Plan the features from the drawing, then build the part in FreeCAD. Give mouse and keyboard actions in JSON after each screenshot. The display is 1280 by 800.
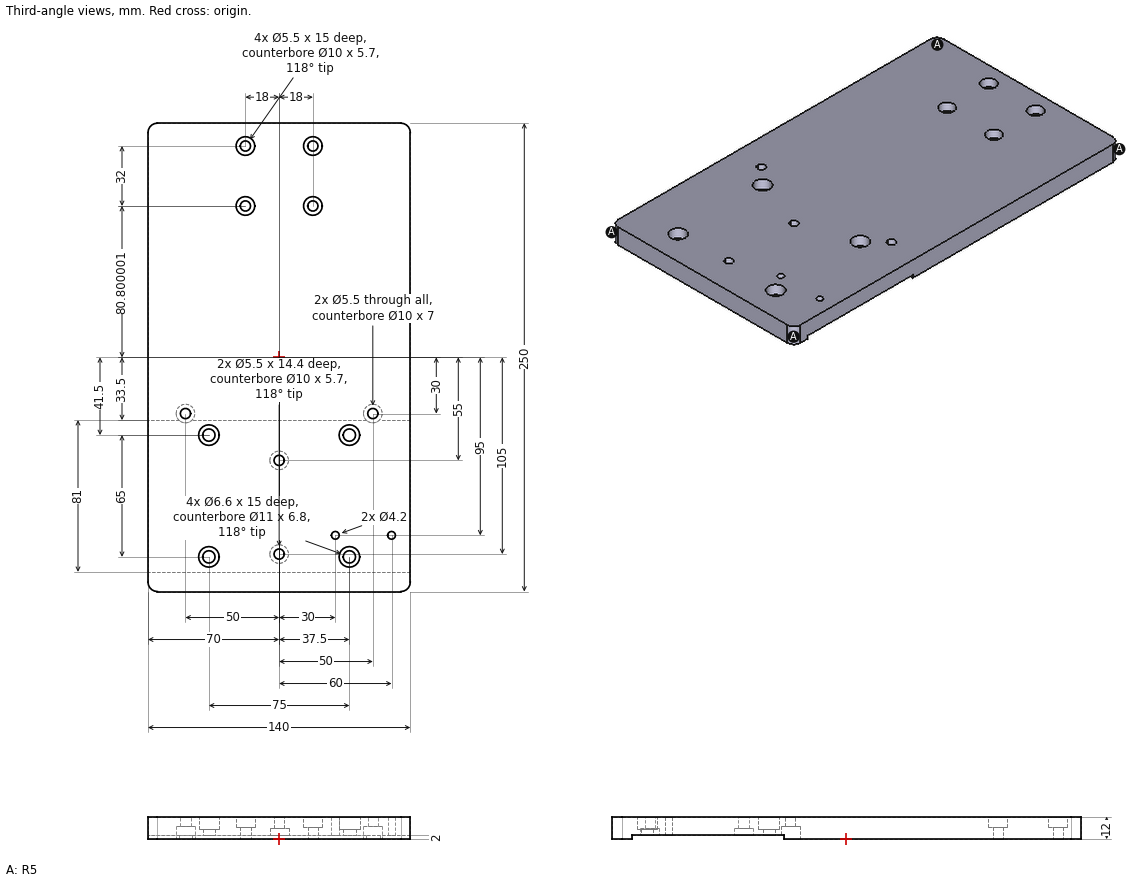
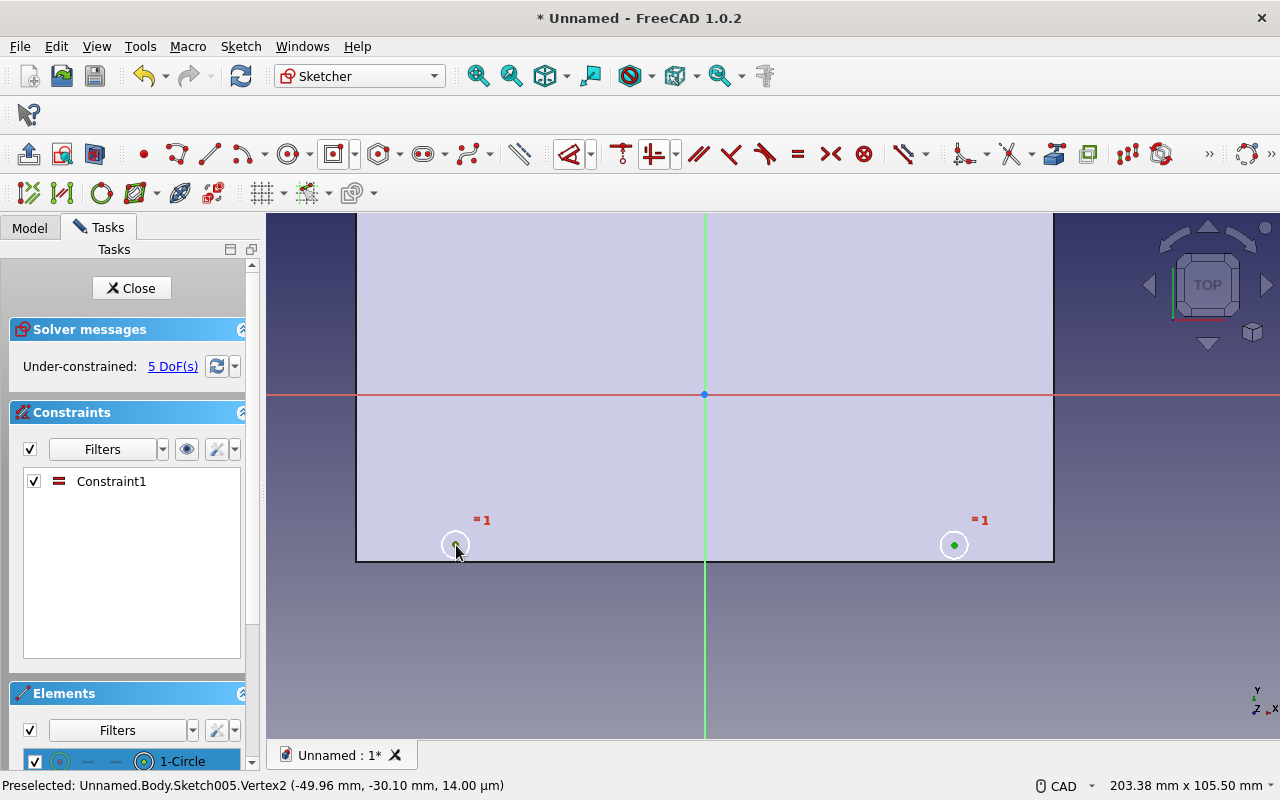
{"action": "key", "text": "h"}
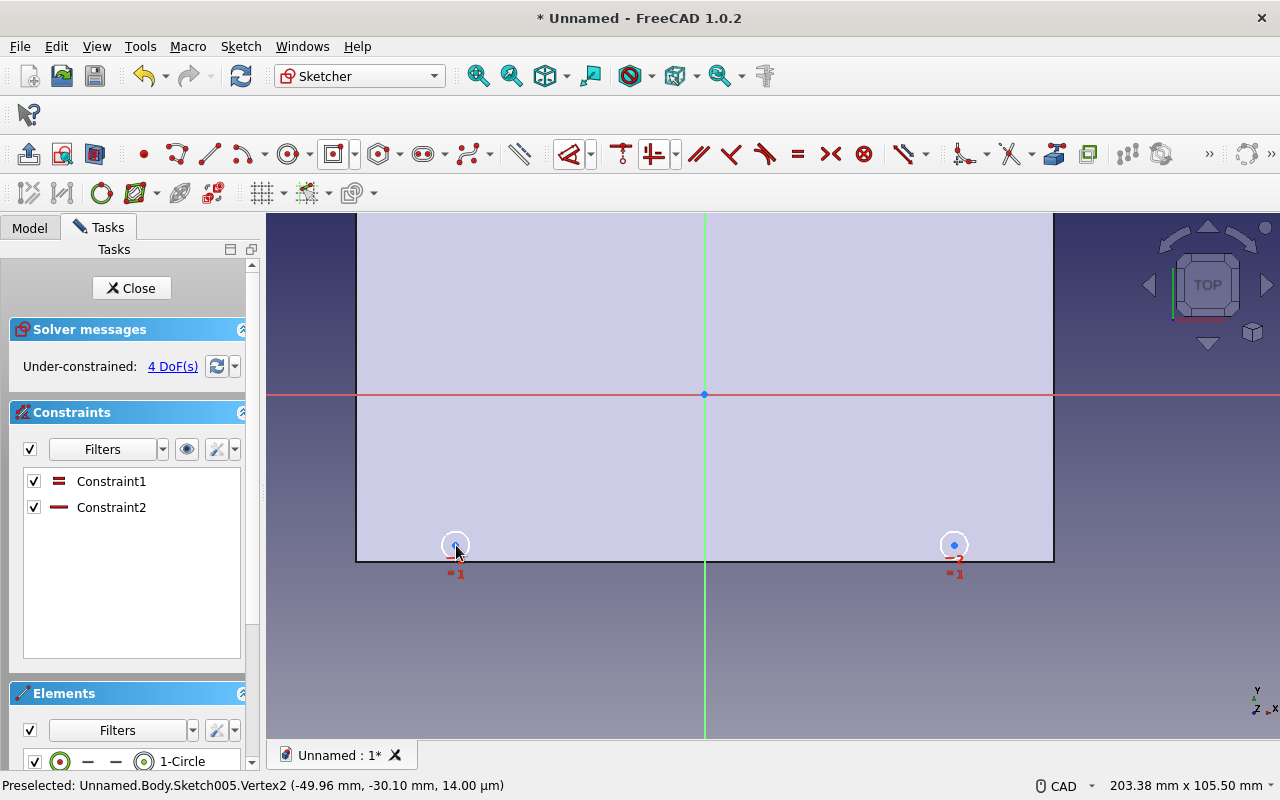
{"action": "scroll", "coordinate": [964, 535], "scroll_direction": "up", "scroll_amount": 2}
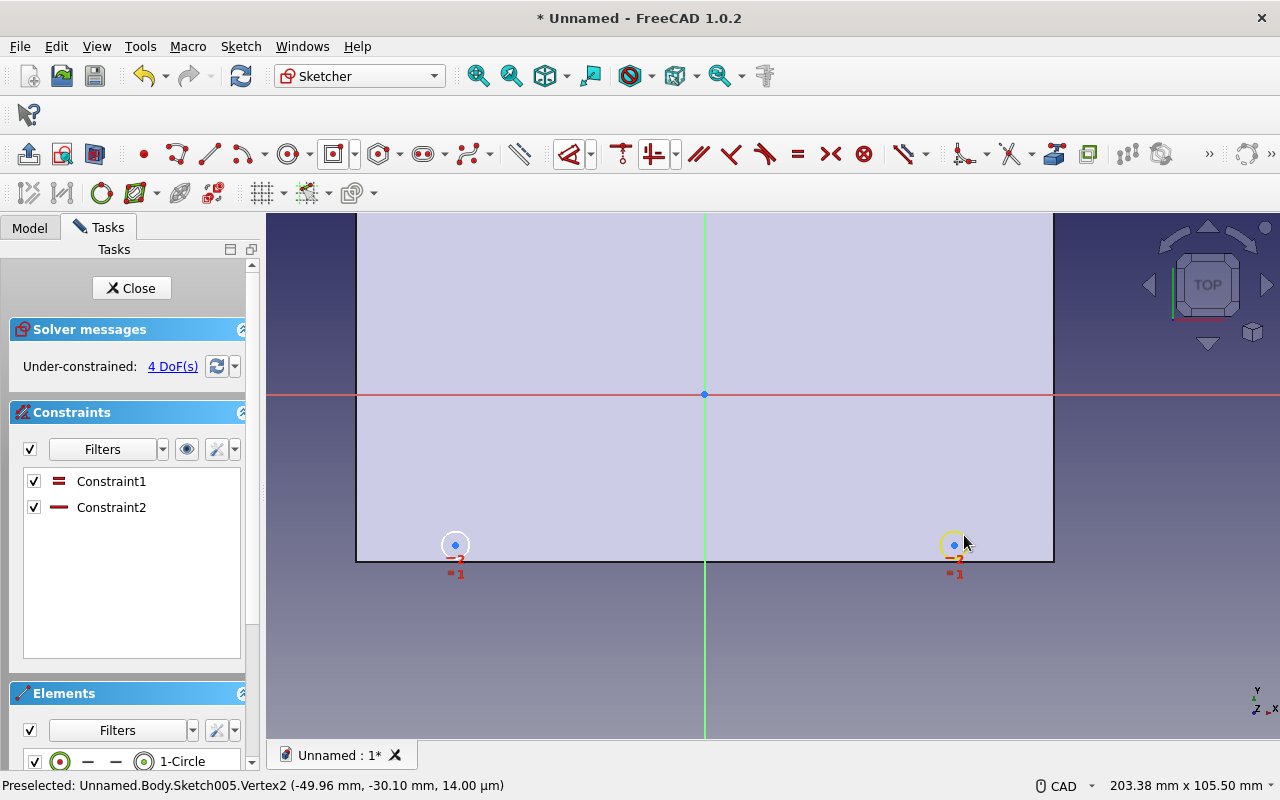
{"action": "left_click", "coordinate": [963, 535]}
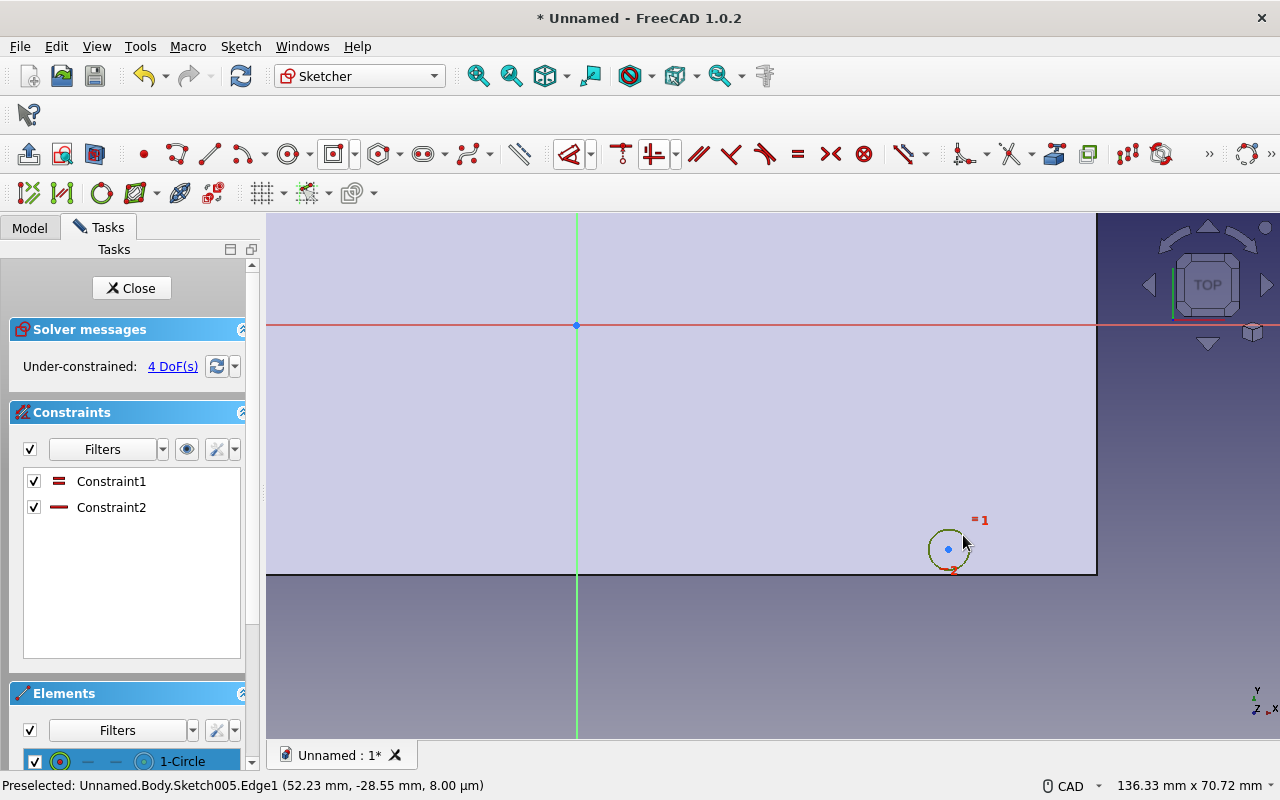
{"action": "key", "text": "k o"}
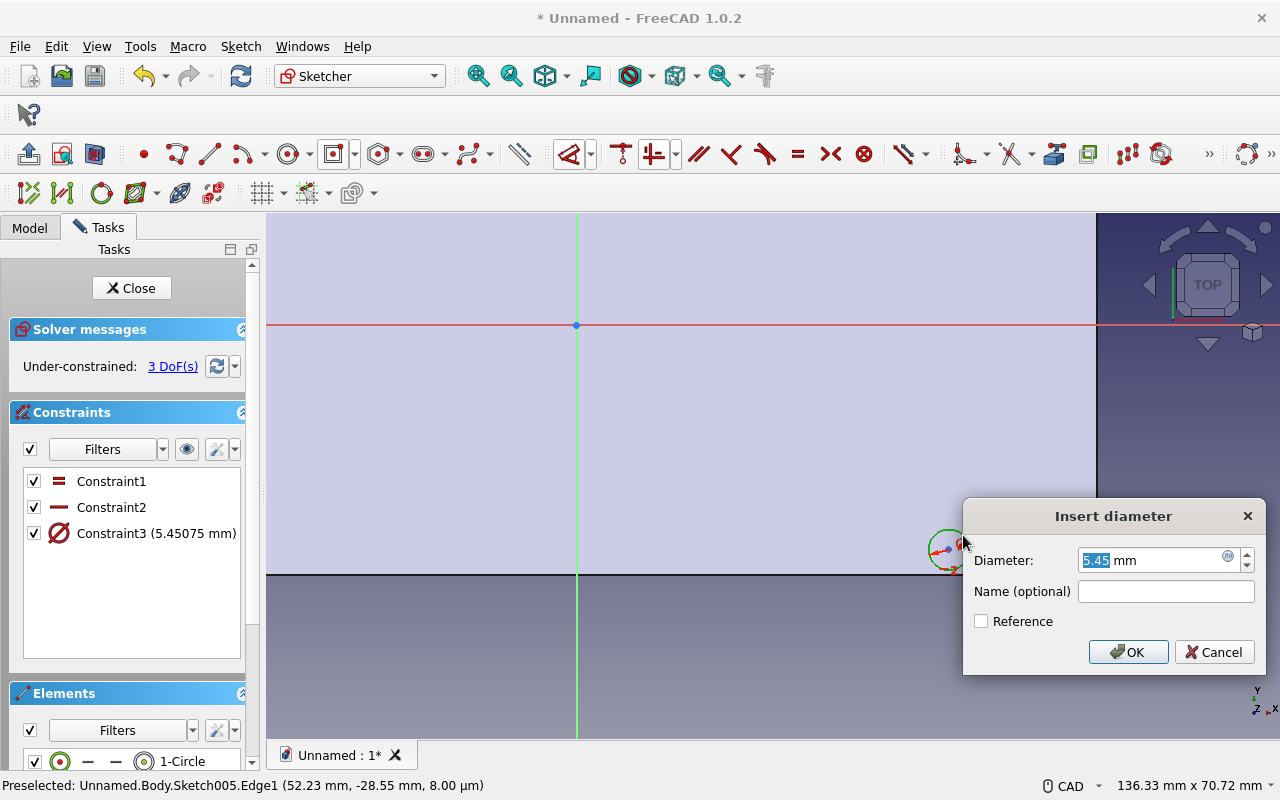
{"action": "type", "text": "5.5"}
{"action": "key", "text": "Return"}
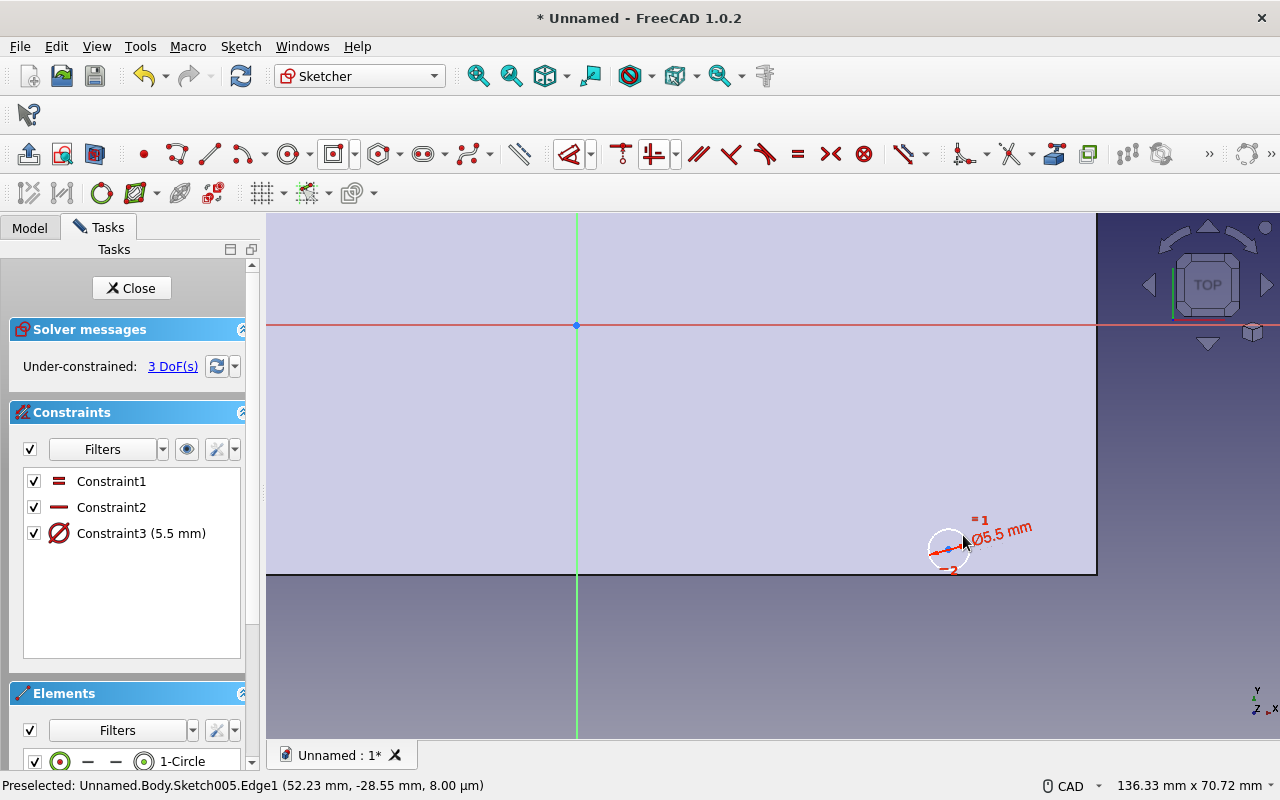
{"action": "left_click", "coordinate": [949, 550]}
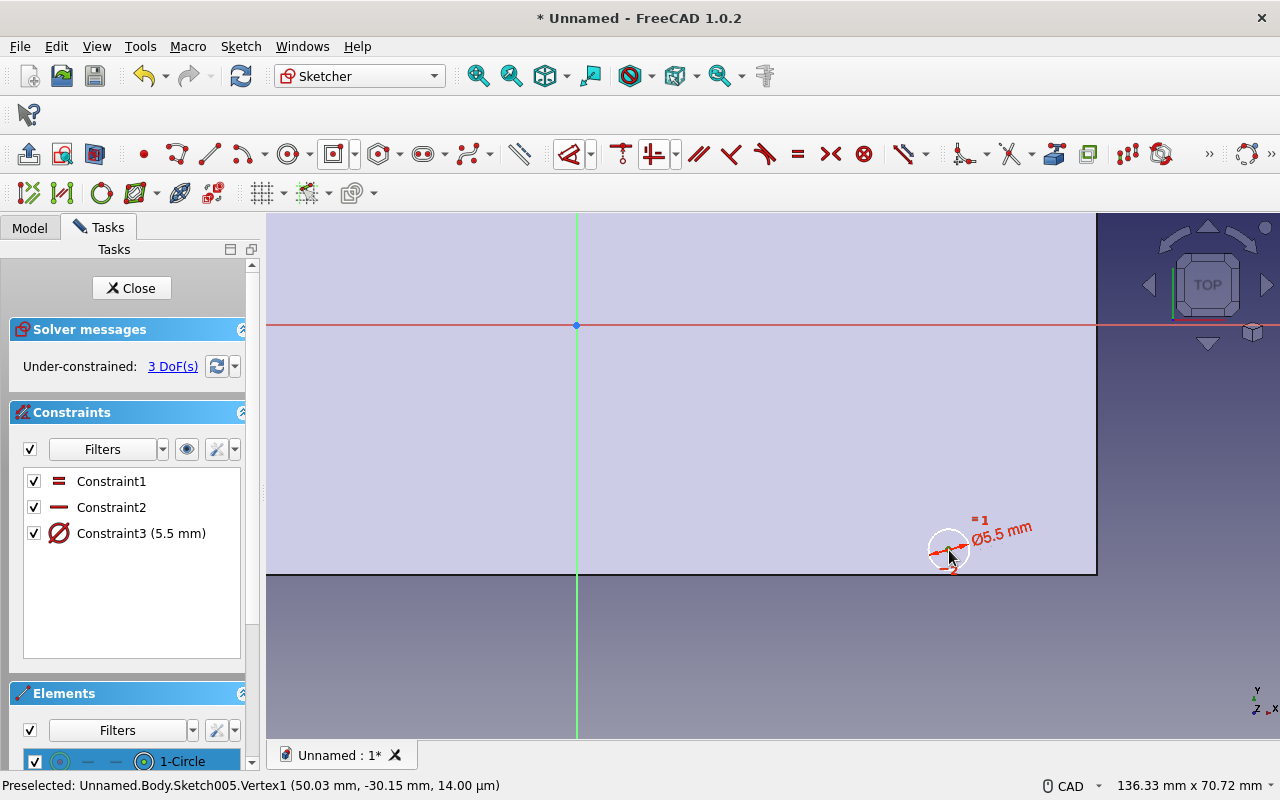
{"action": "left_click", "coordinate": [590, 154]}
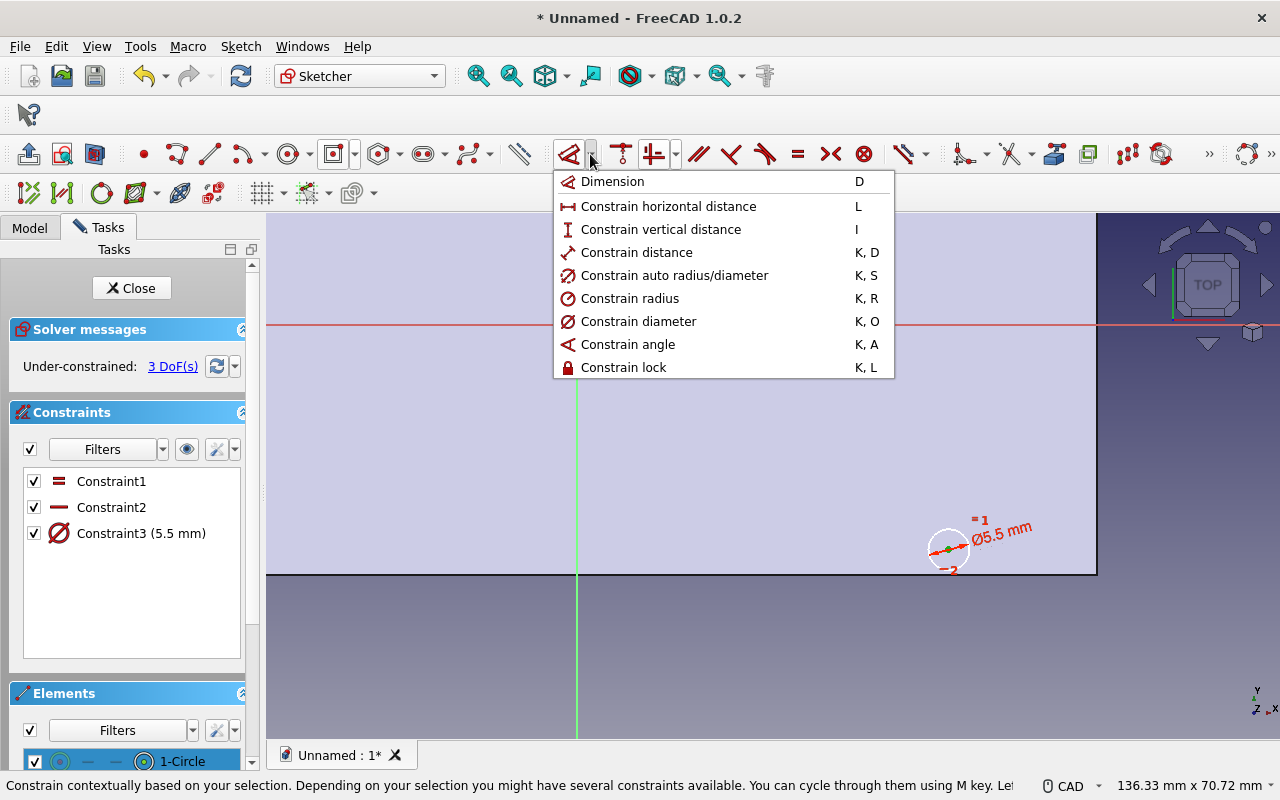
{"action": "left_click", "coordinate": [724, 206]}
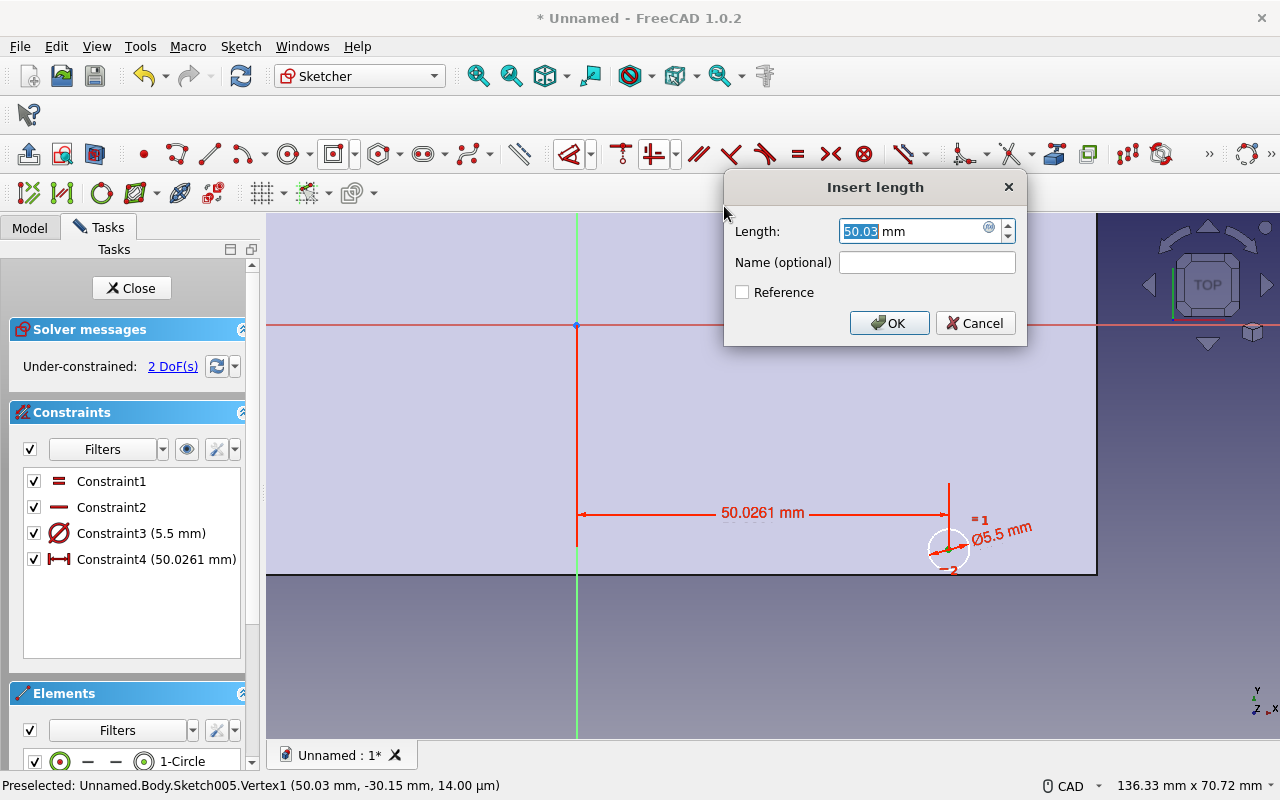
{"action": "type", "text": "50"}
{"action": "key", "text": "Return"}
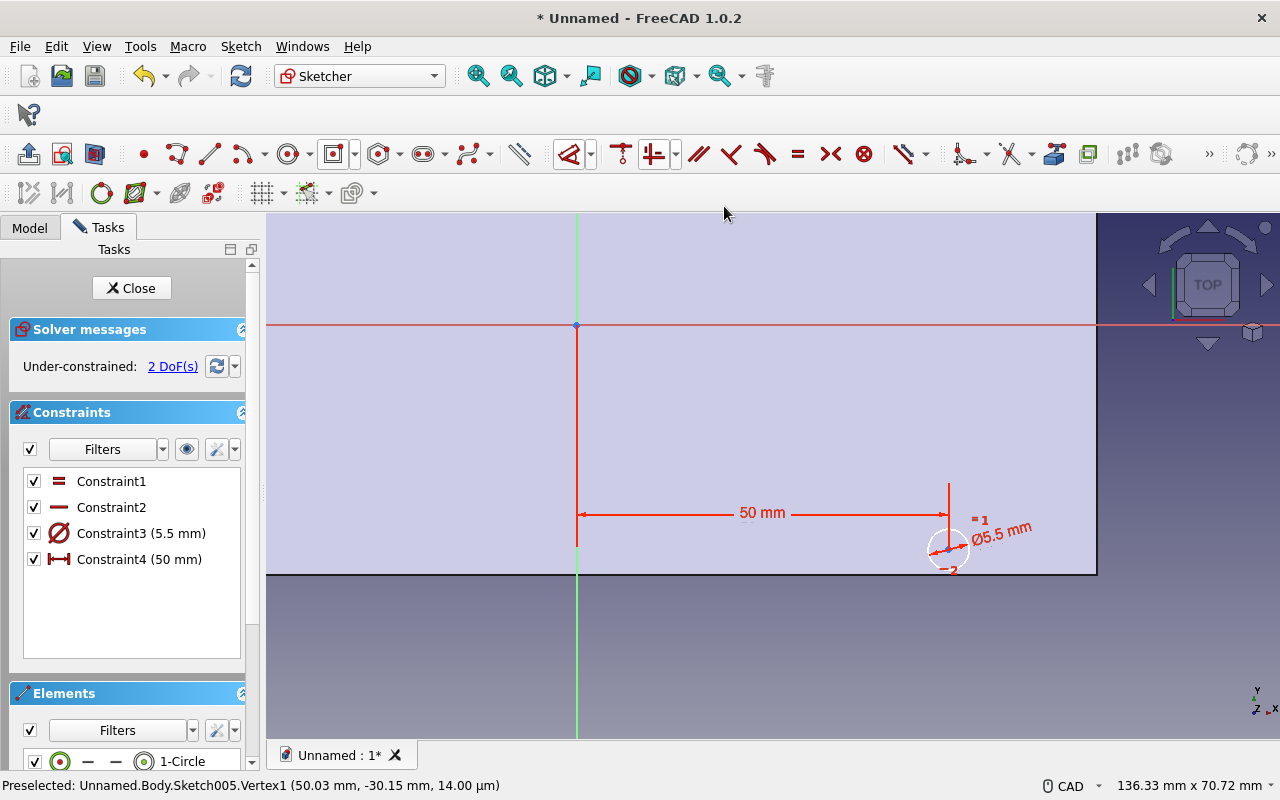
{"action": "left_click", "coordinate": [949, 550]}